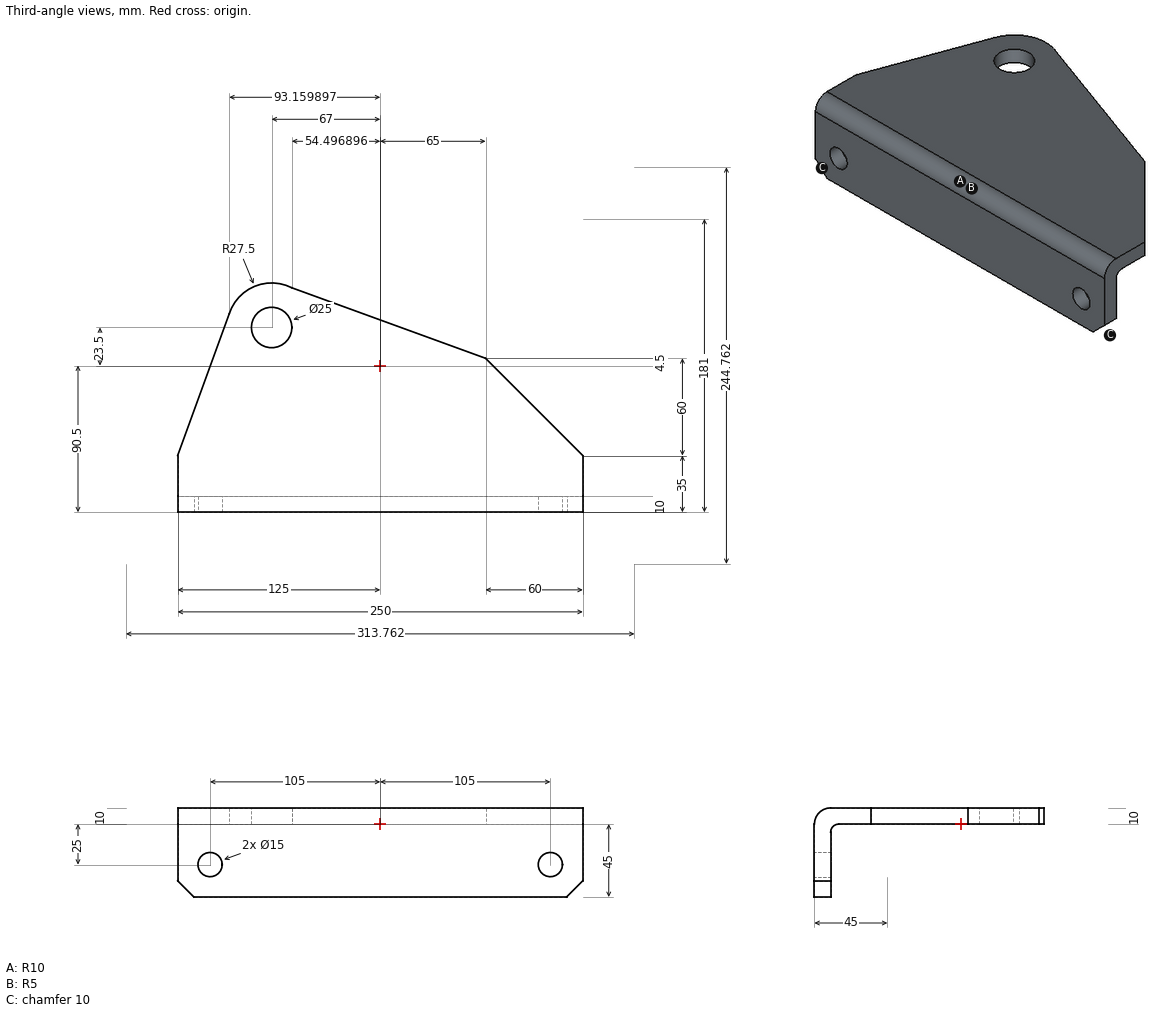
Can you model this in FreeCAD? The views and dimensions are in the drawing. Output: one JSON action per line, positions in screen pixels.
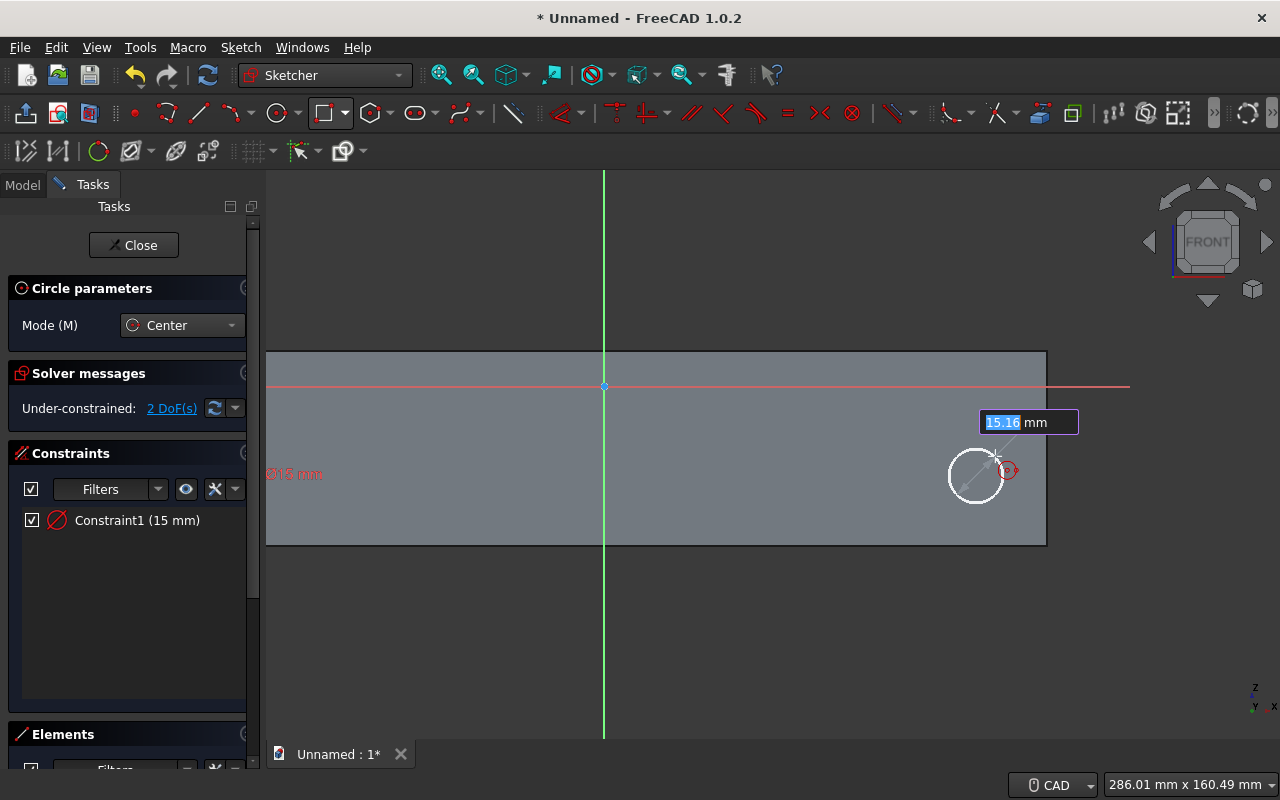
{"action": "type", "text": "15"}
{"action": "key", "text": "Return"}
{"action": "key", "text": "Escape"}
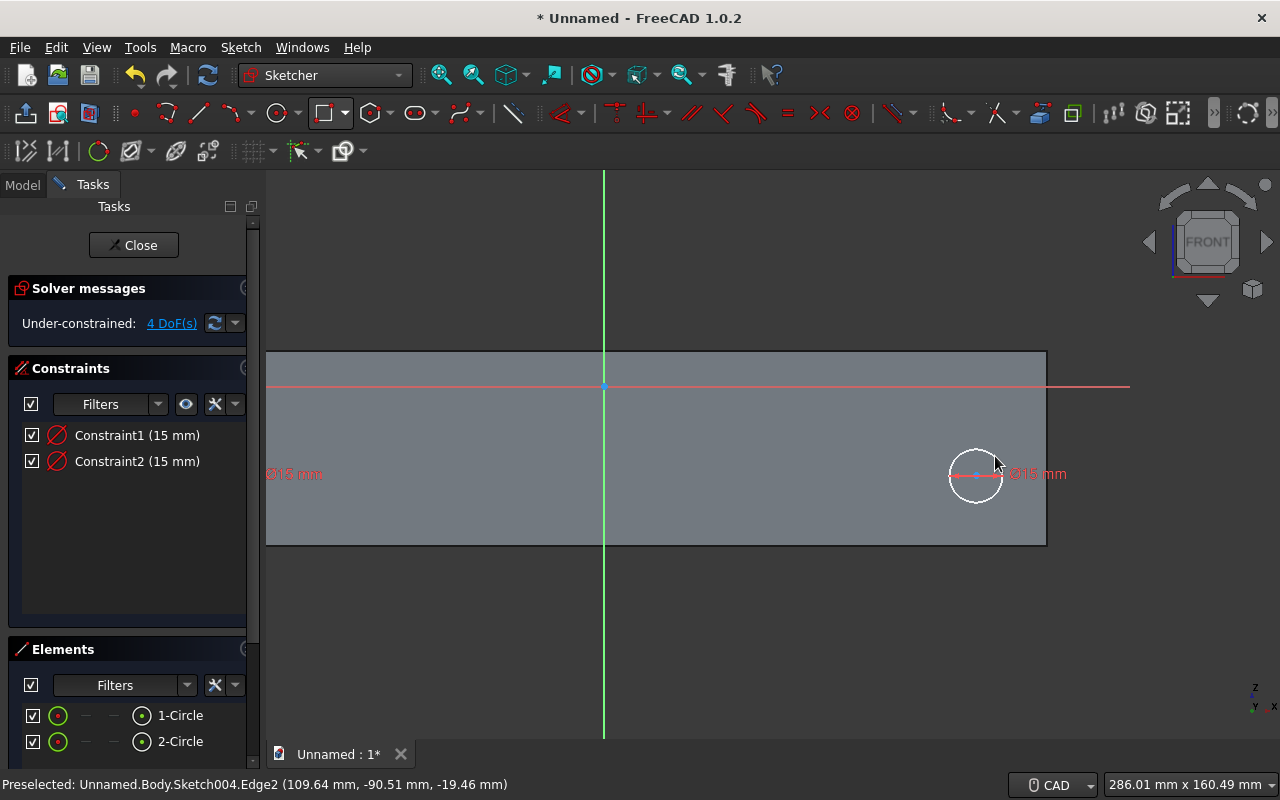
{"action": "scroll", "coordinate": [908, 476], "scroll_direction": "down", "scroll_amount": 2}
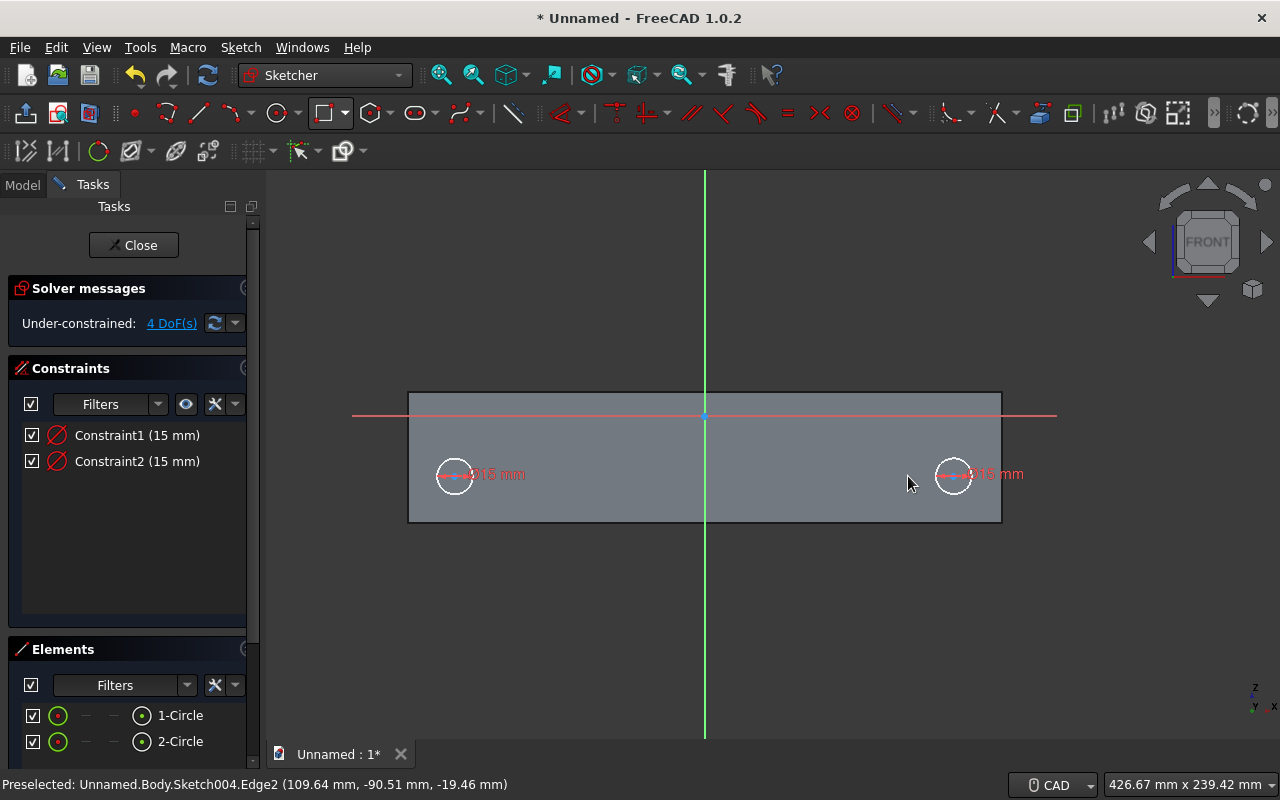
{"action": "left_click", "coordinate": [455, 476]}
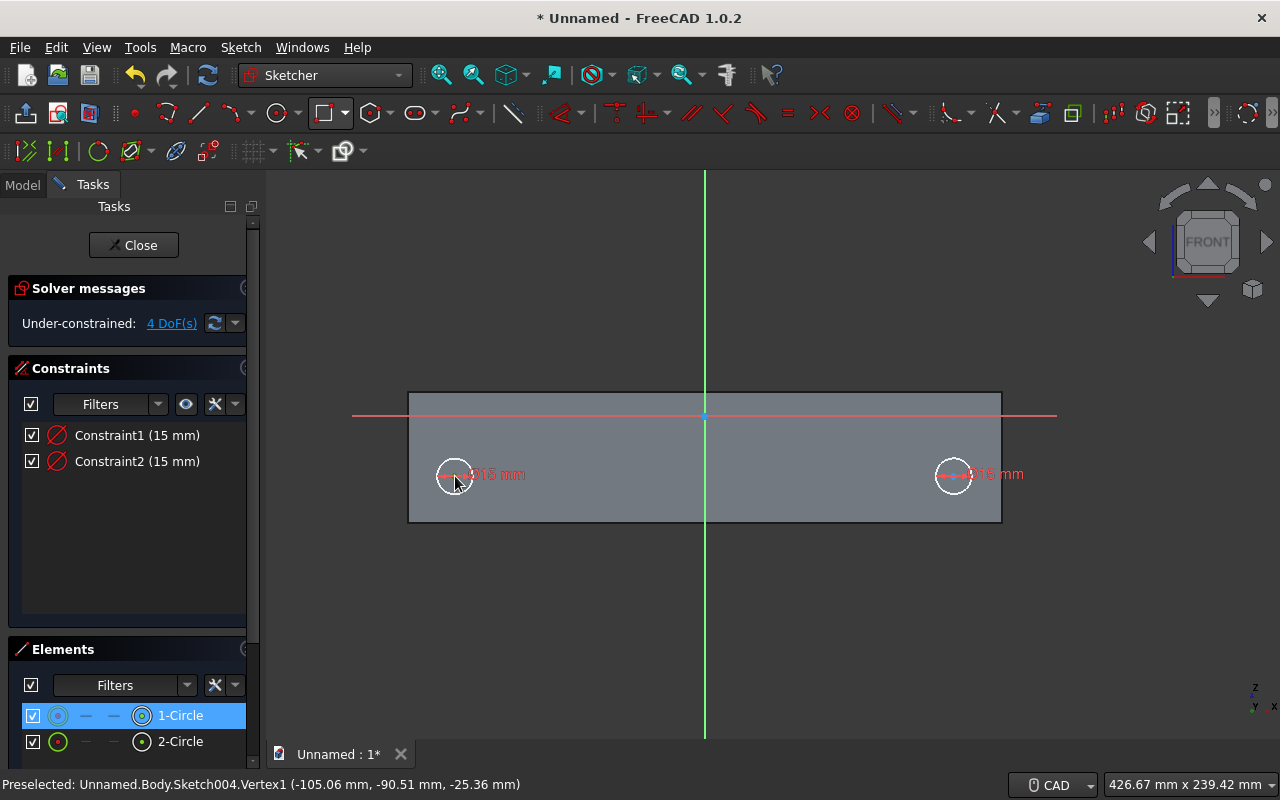
{"action": "left_click", "coordinate": [954, 476]}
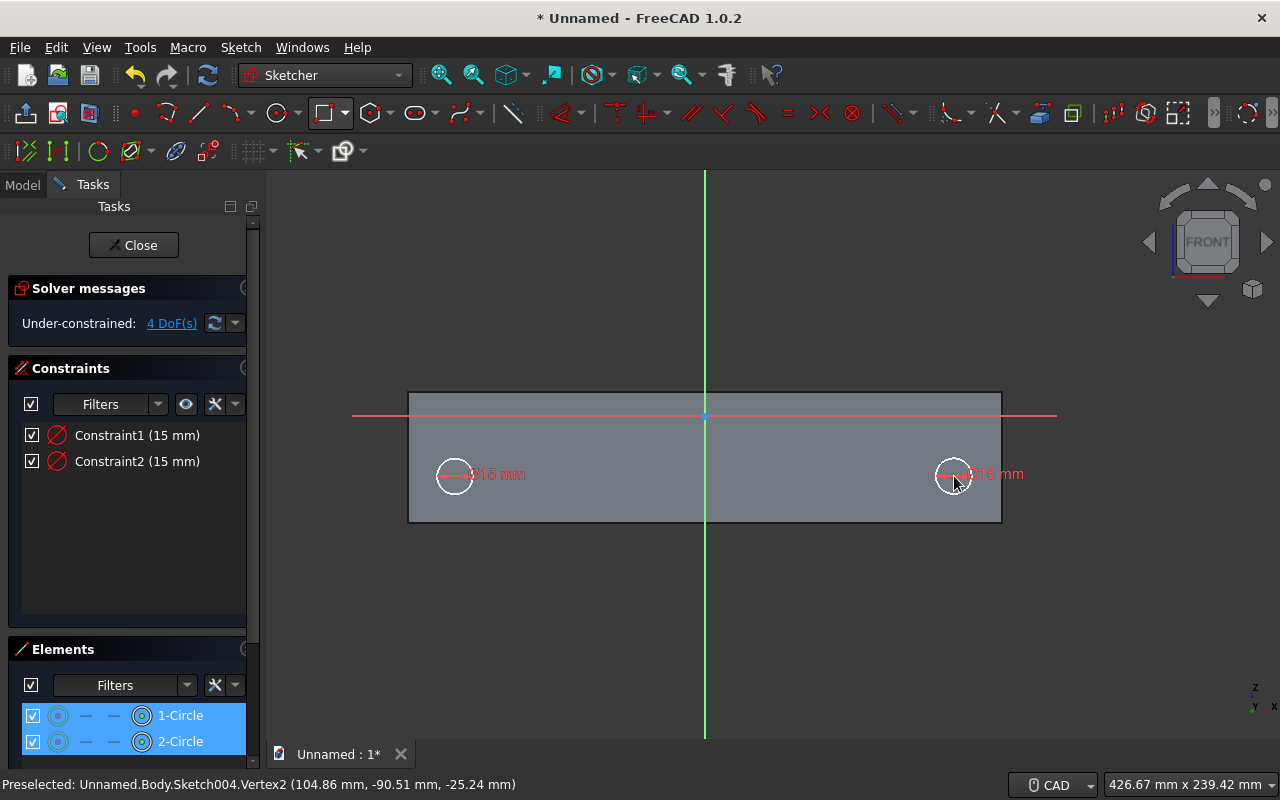
{"action": "key", "text": "h"}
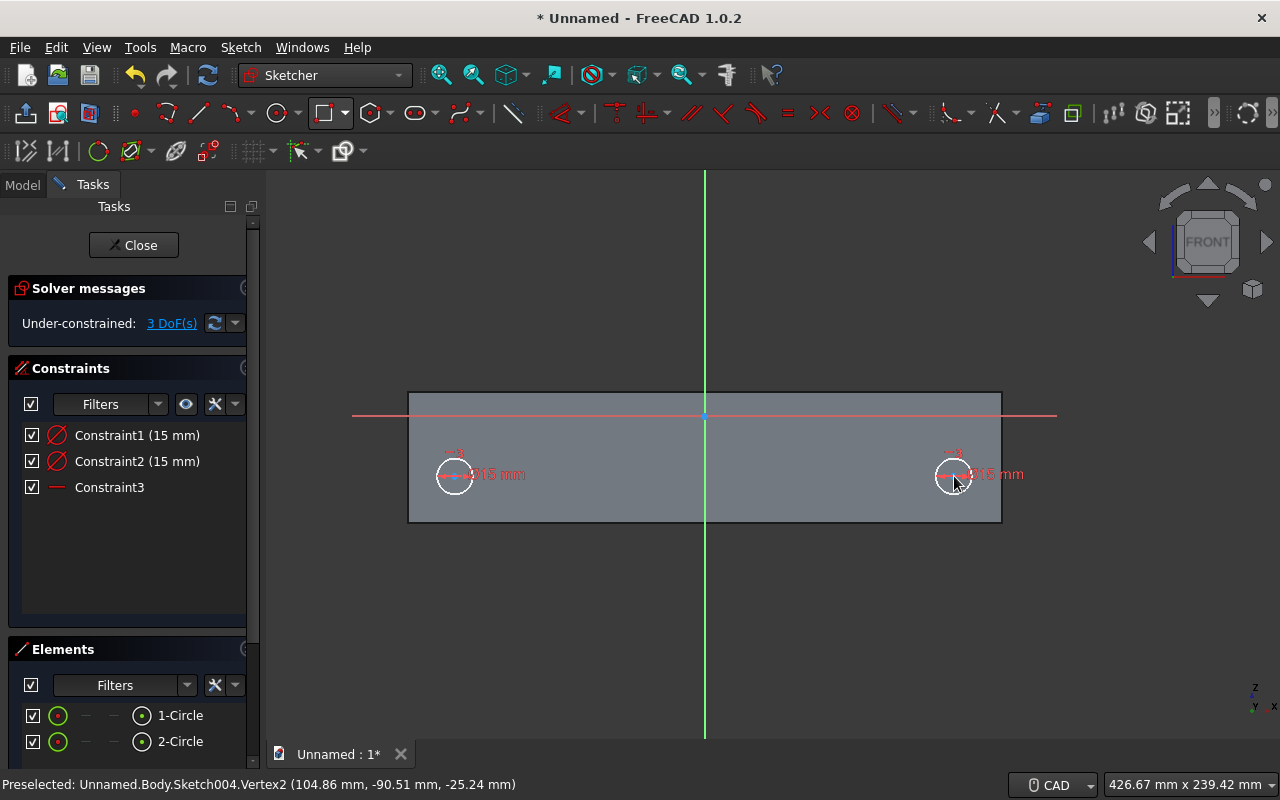
{"action": "left_click", "coordinate": [560, 114]}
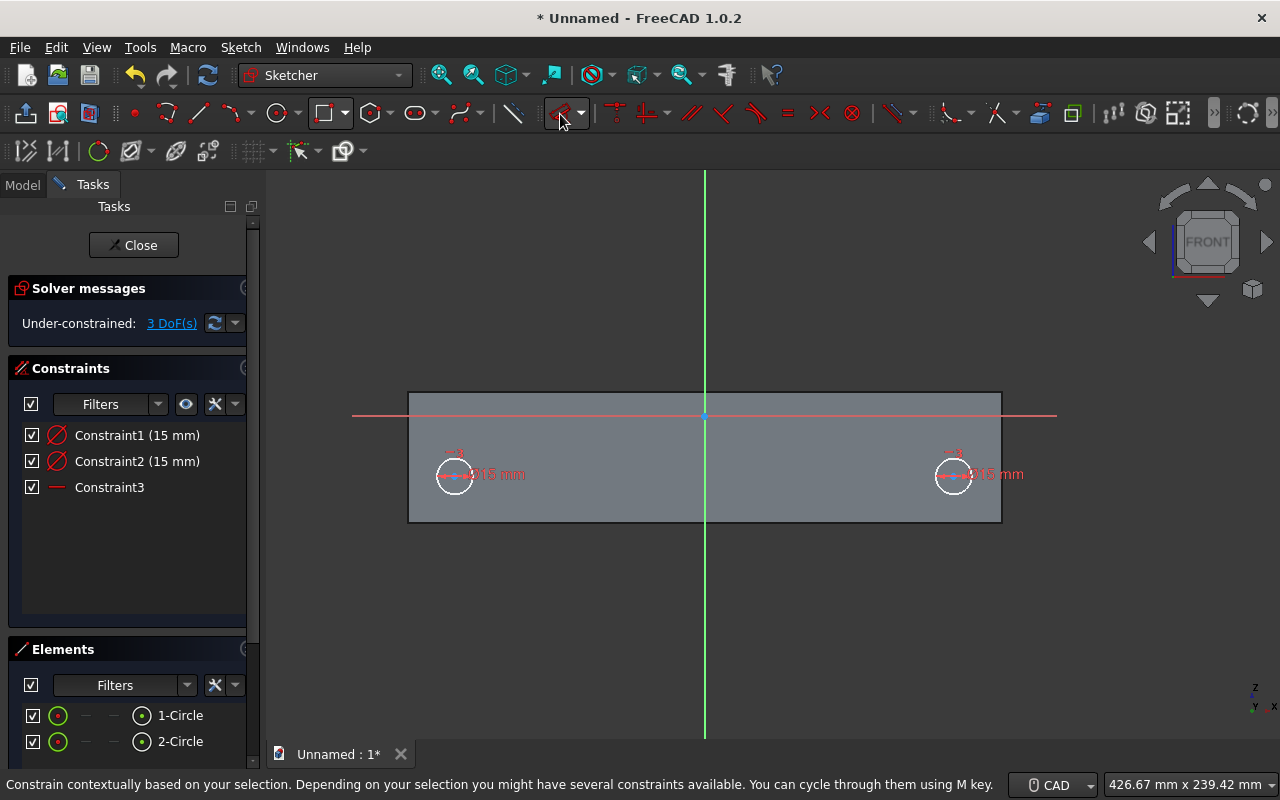
{"action": "left_click", "coordinate": [455, 476]}
{"action": "left_click", "coordinate": [421, 446]}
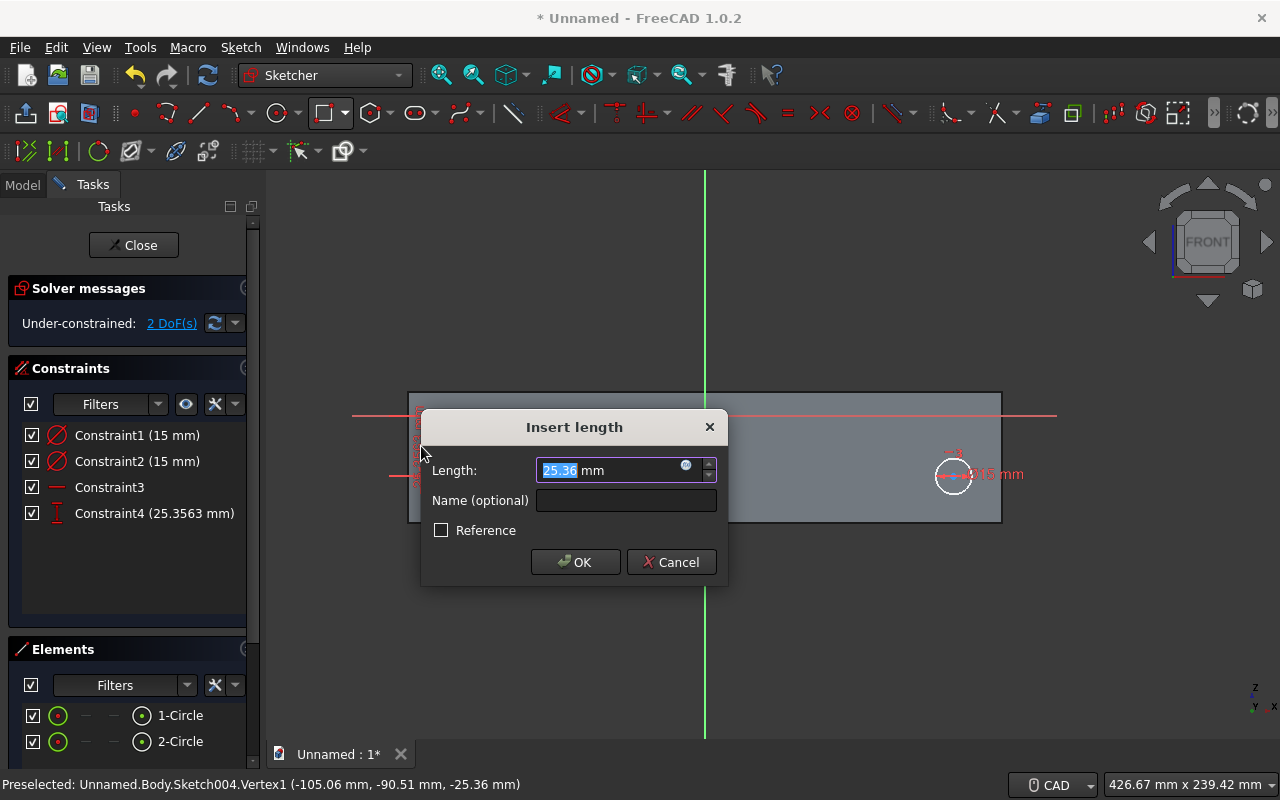
{"action": "type", "text": "25"}
{"action": "key", "text": "Return"}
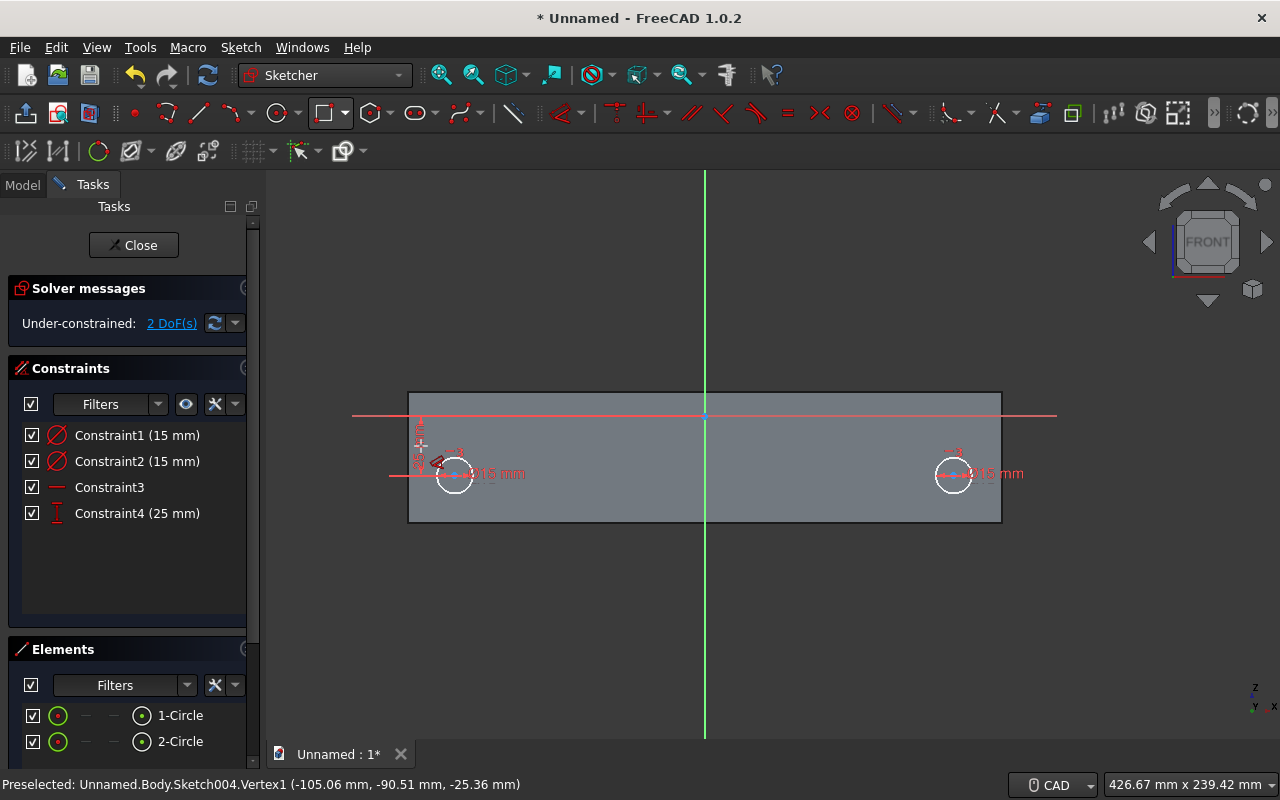
{"action": "left_click", "coordinate": [455, 476]}
{"action": "left_click", "coordinate": [580, 382]}